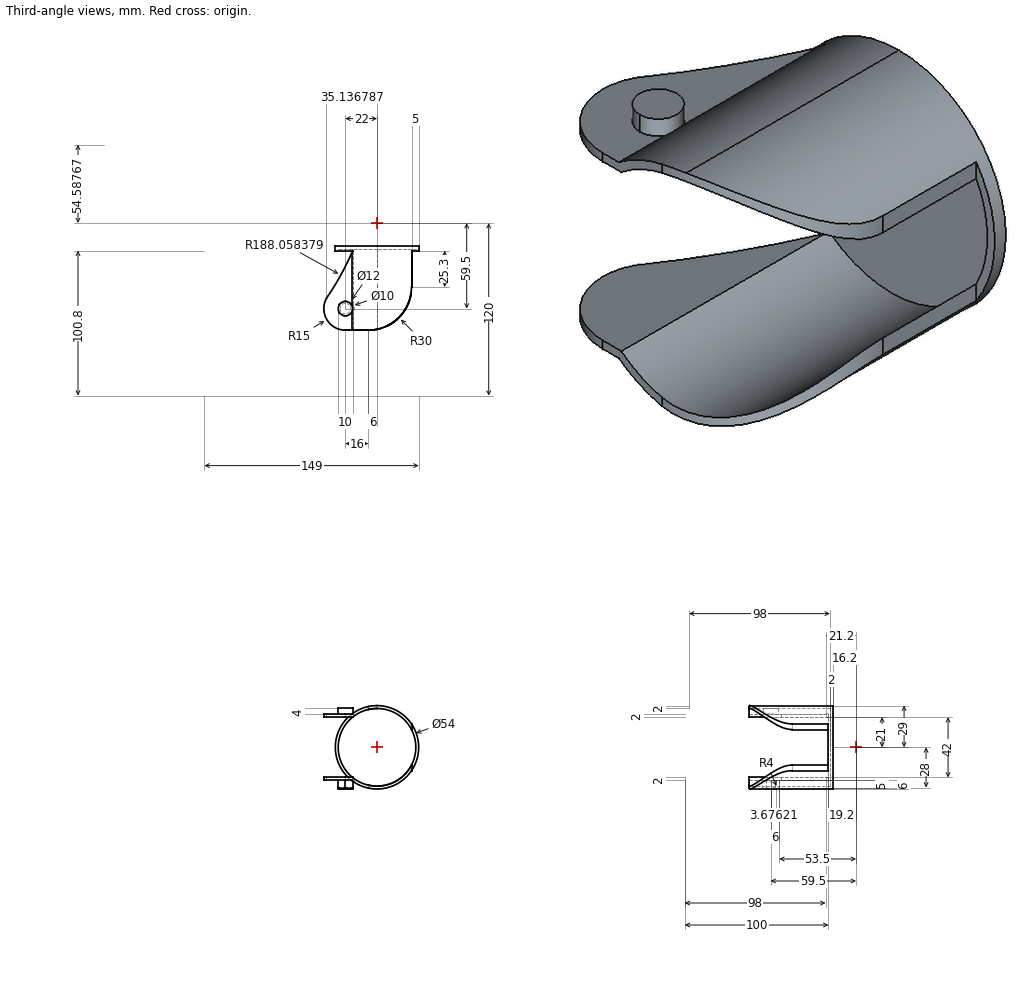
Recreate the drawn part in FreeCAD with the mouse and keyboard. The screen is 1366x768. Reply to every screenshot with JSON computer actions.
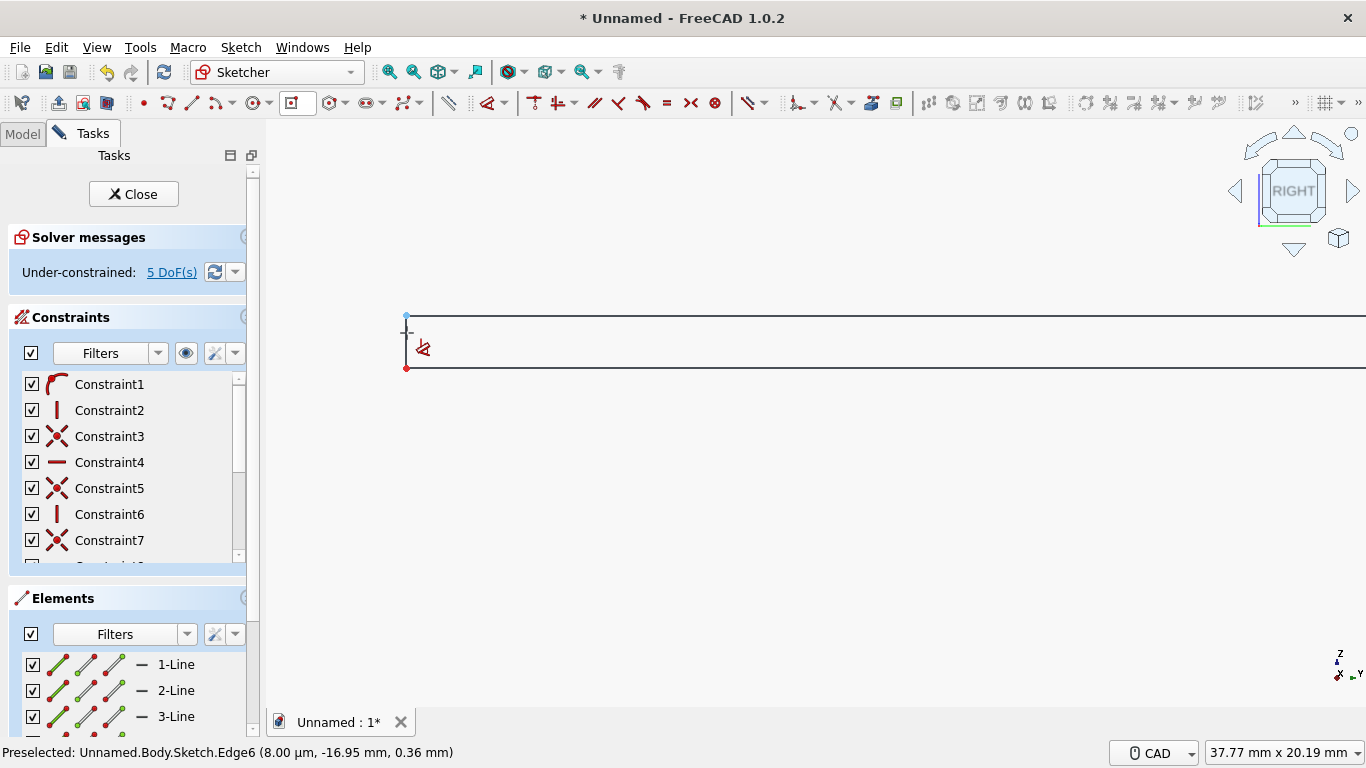
{"action": "left_click", "coordinate": [406, 332]}
{"action": "left_click", "coordinate": [372, 342]}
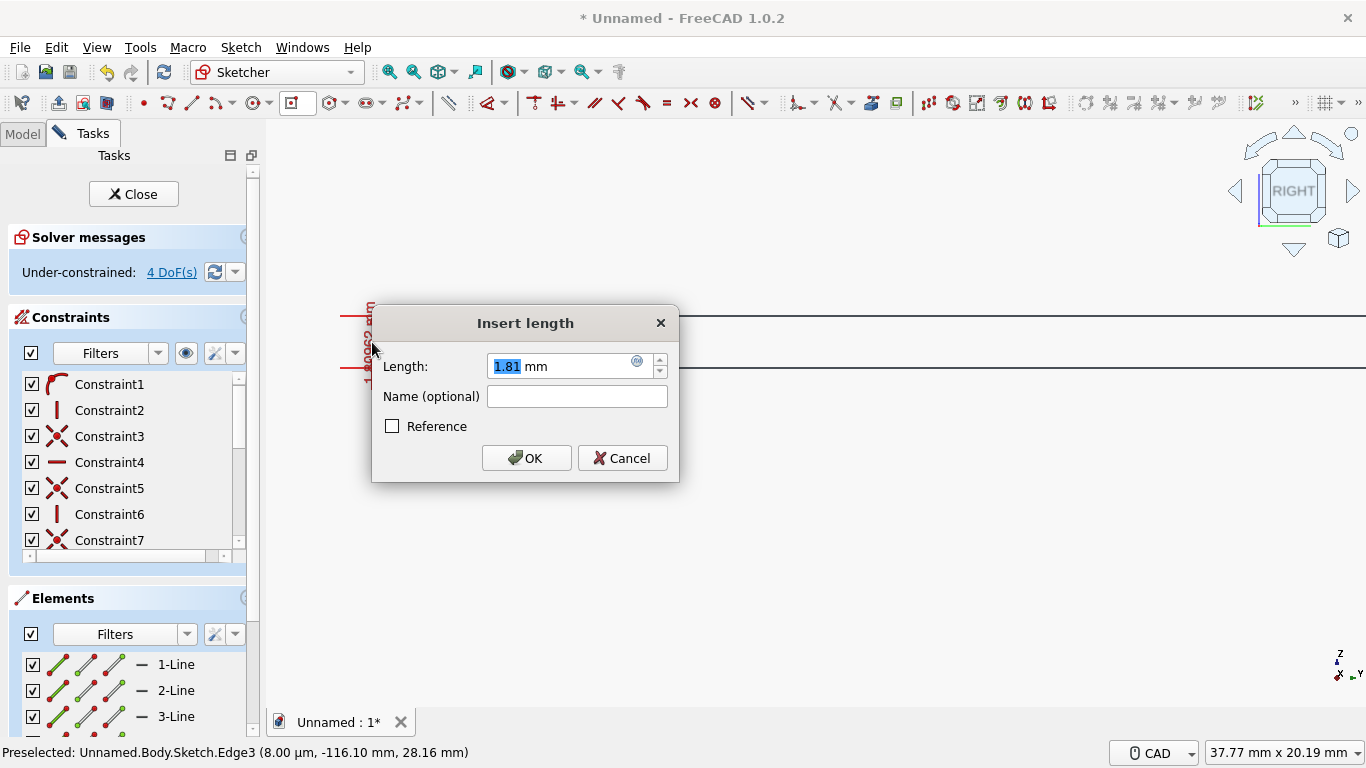
{"action": "type", "text": "2"}
{"action": "key", "text": "Return"}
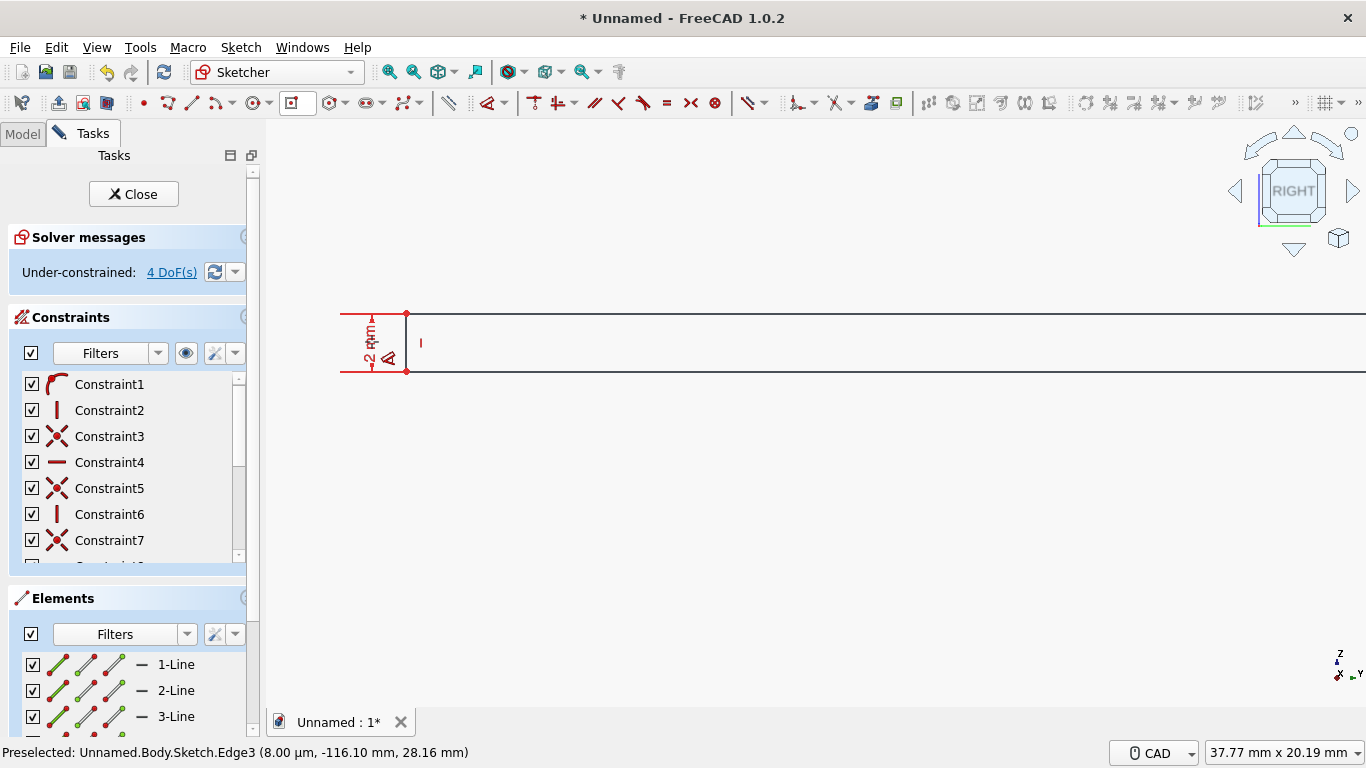
{"action": "scroll", "coordinate": [406, 333], "scroll_direction": "down", "scroll_amount": 8}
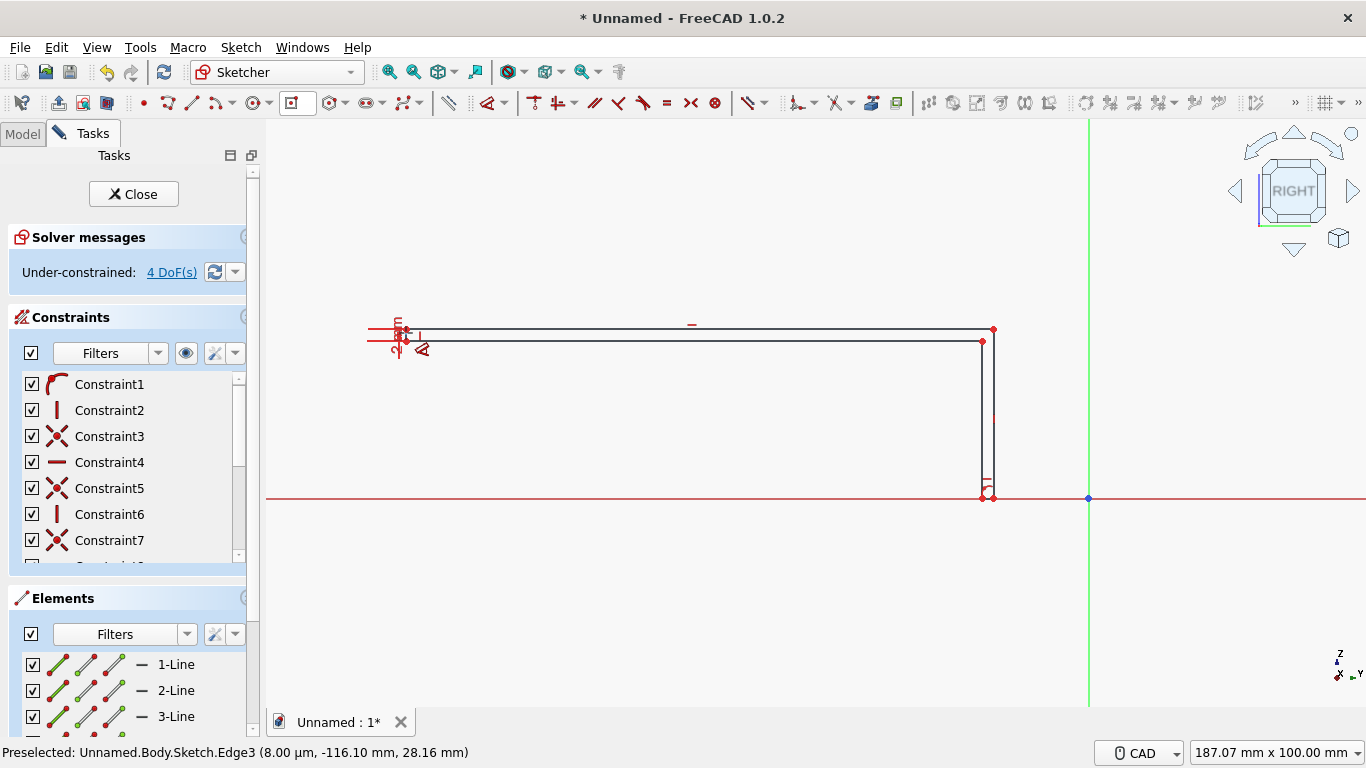
{"action": "scroll", "coordinate": [986, 499], "scroll_direction": "up", "scroll_amount": 7}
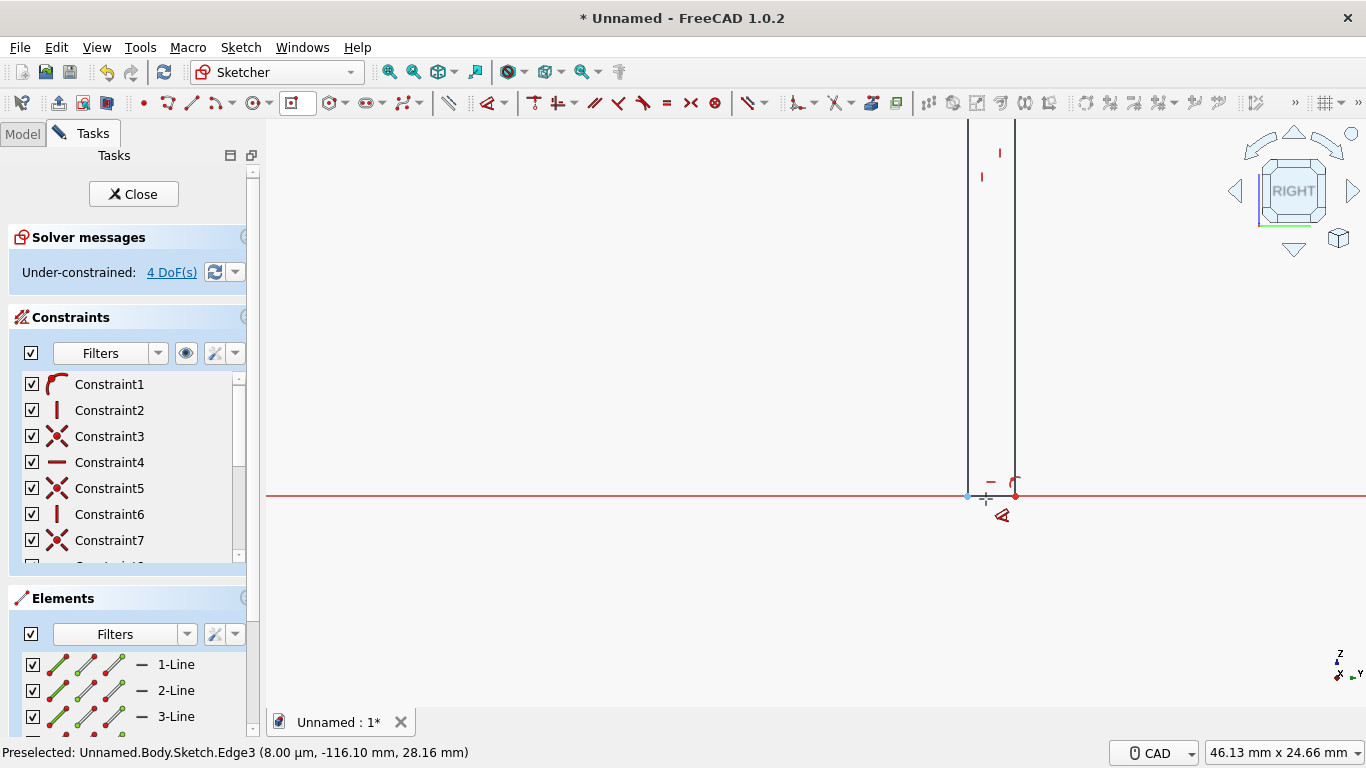
{"action": "left_click", "coordinate": [982, 496]}
{"action": "left_click", "coordinate": [992, 530]}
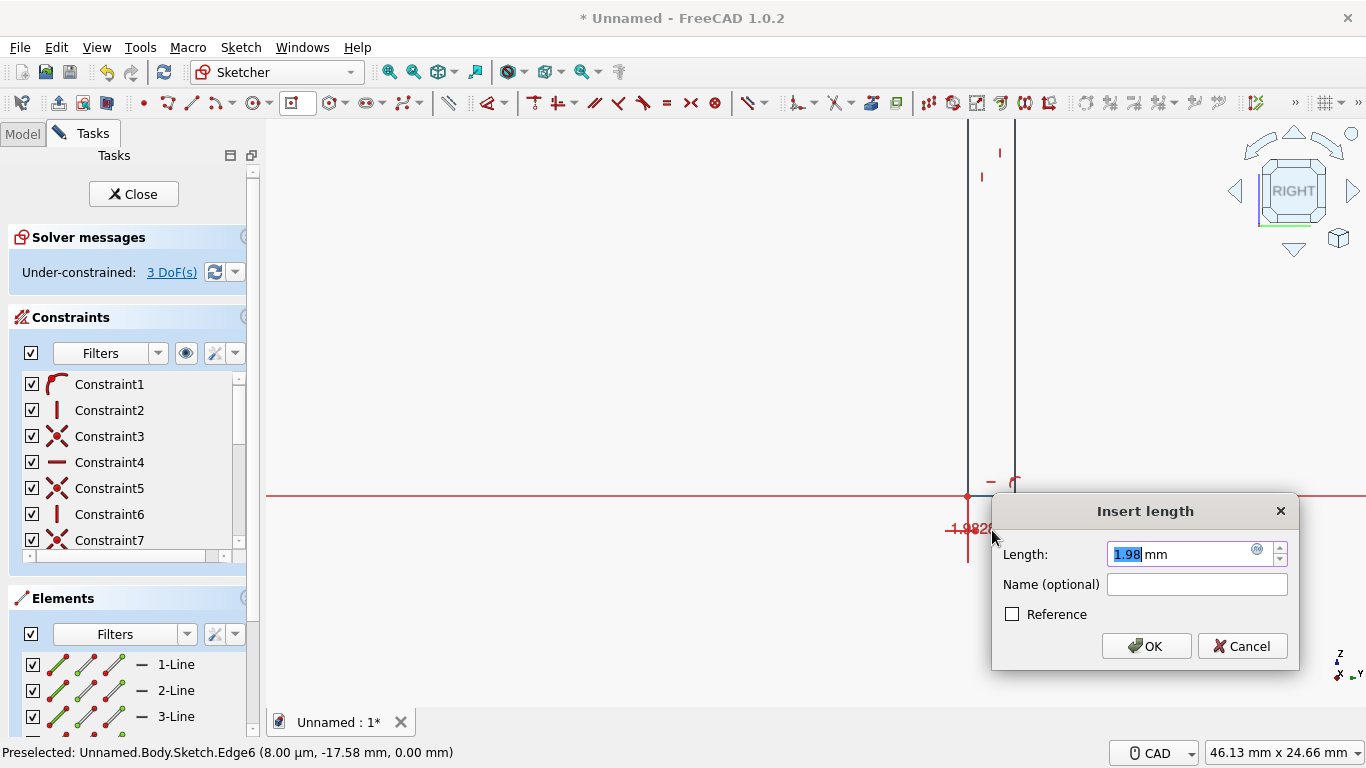
{"action": "type", "text": "2"}
{"action": "key", "text": "Return"}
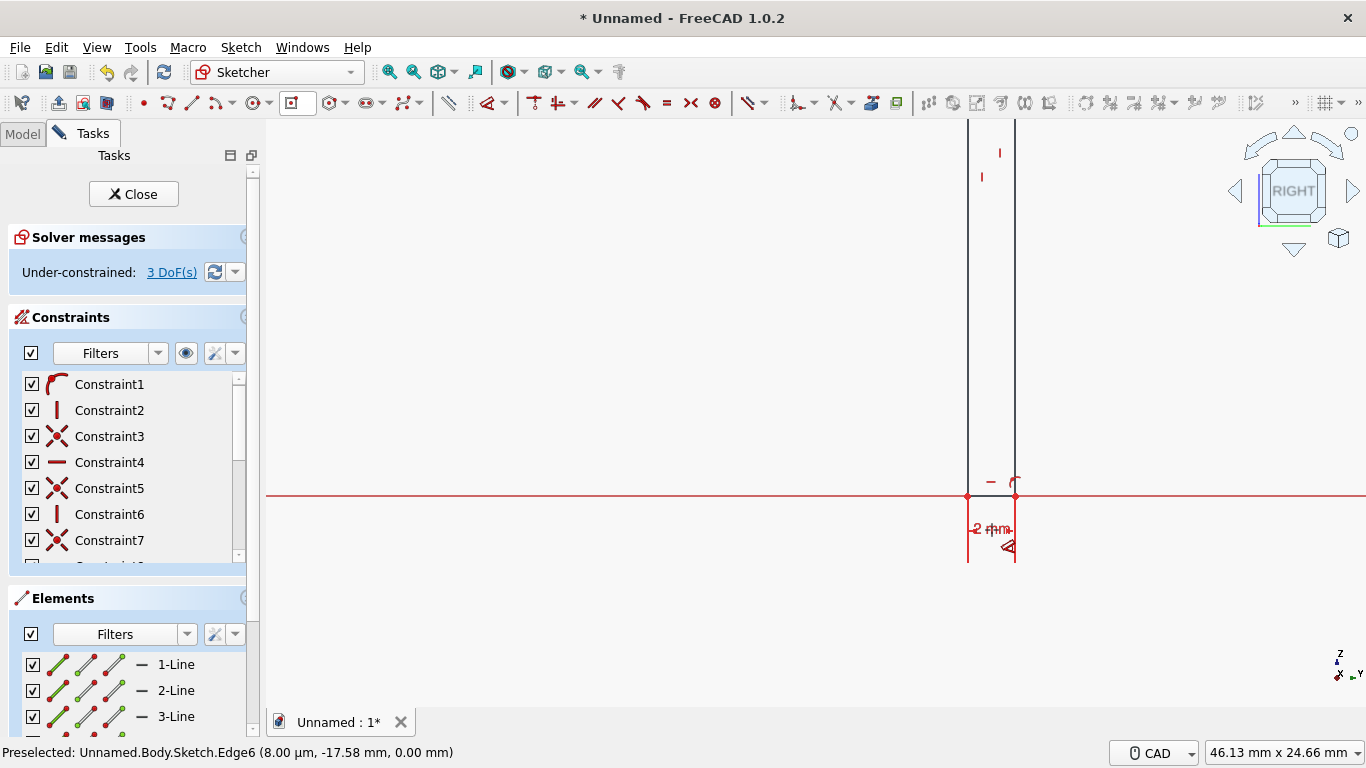
{"action": "scroll", "coordinate": [987, 499], "scroll_direction": "down", "scroll_amount": 7}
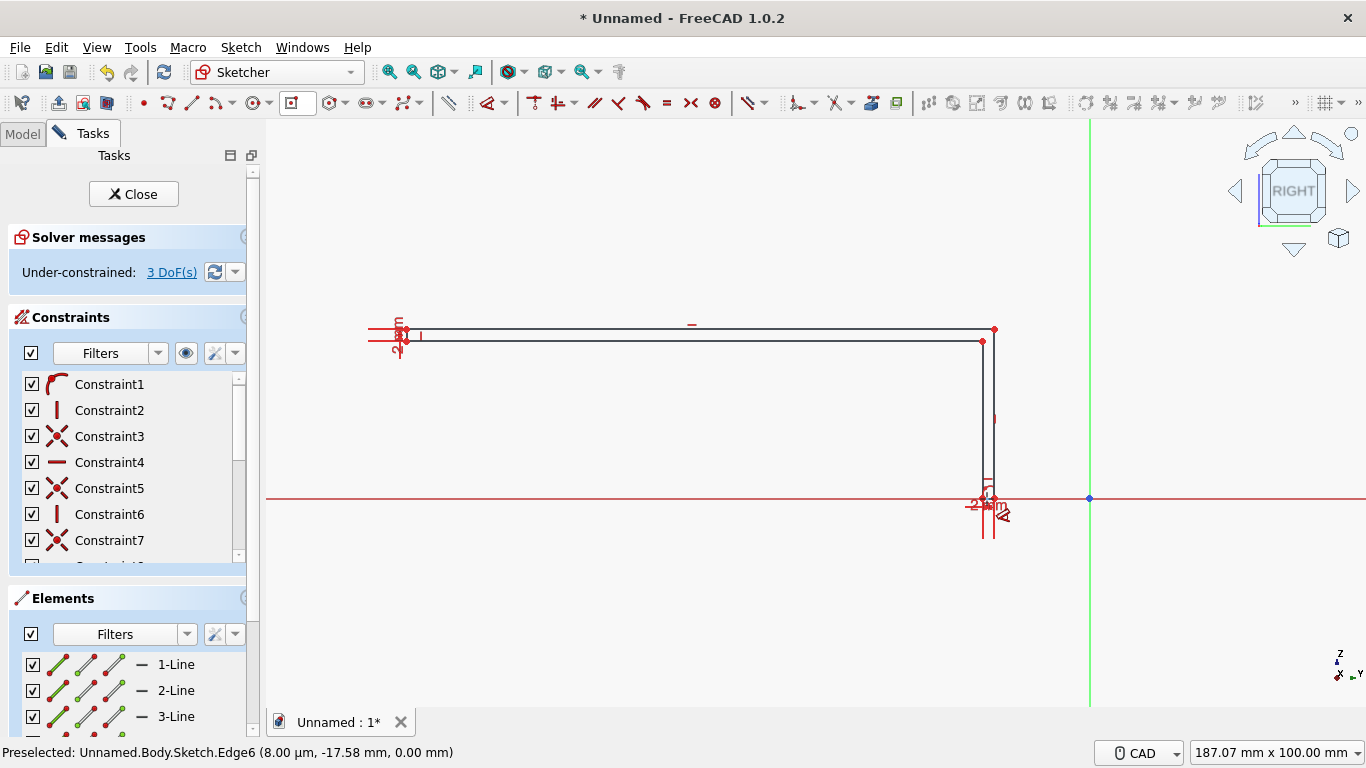
{"action": "left_click", "coordinate": [994, 448]}
{"action": "left_click", "coordinate": [1028, 414]}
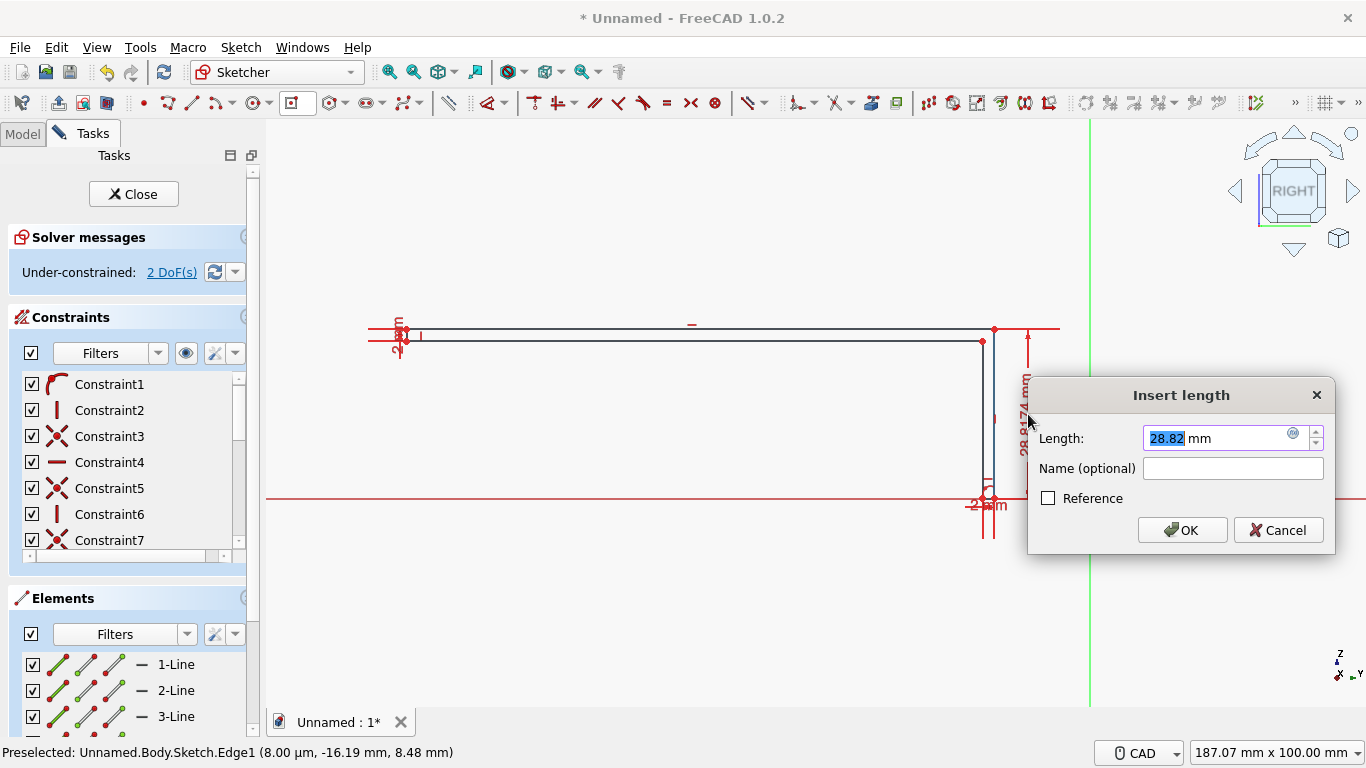
{"action": "type", "text": "29"}
{"action": "key", "text": "Return"}